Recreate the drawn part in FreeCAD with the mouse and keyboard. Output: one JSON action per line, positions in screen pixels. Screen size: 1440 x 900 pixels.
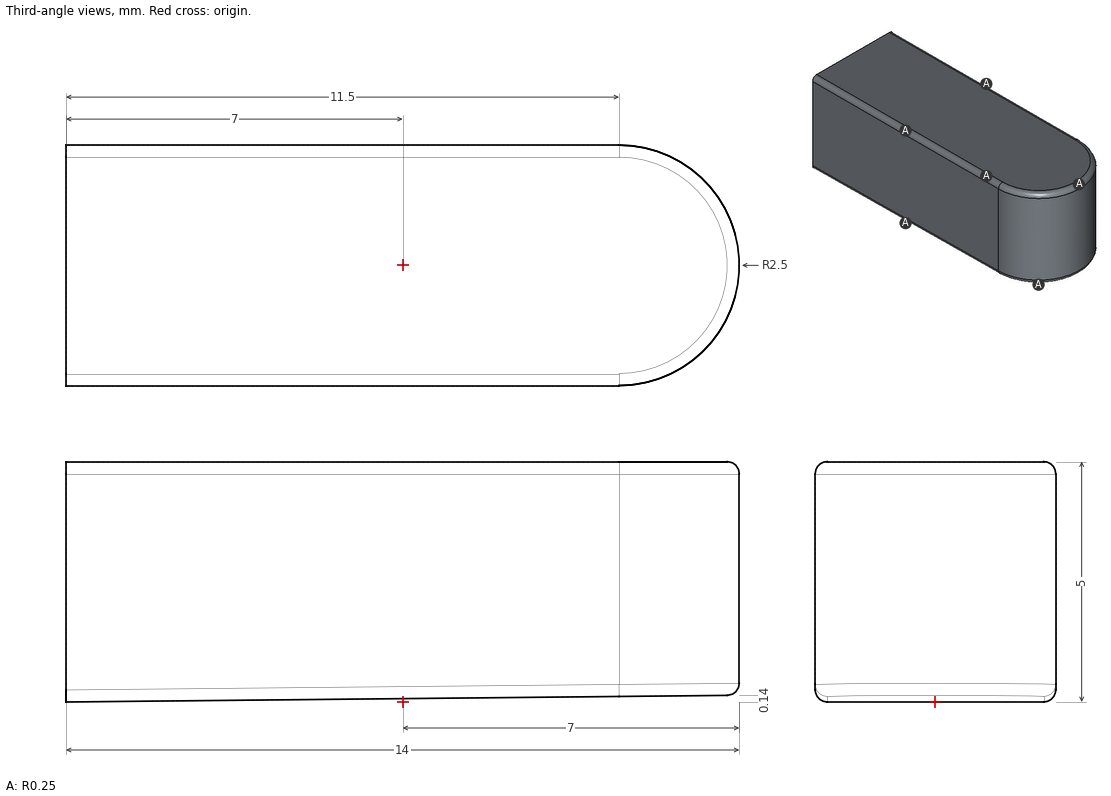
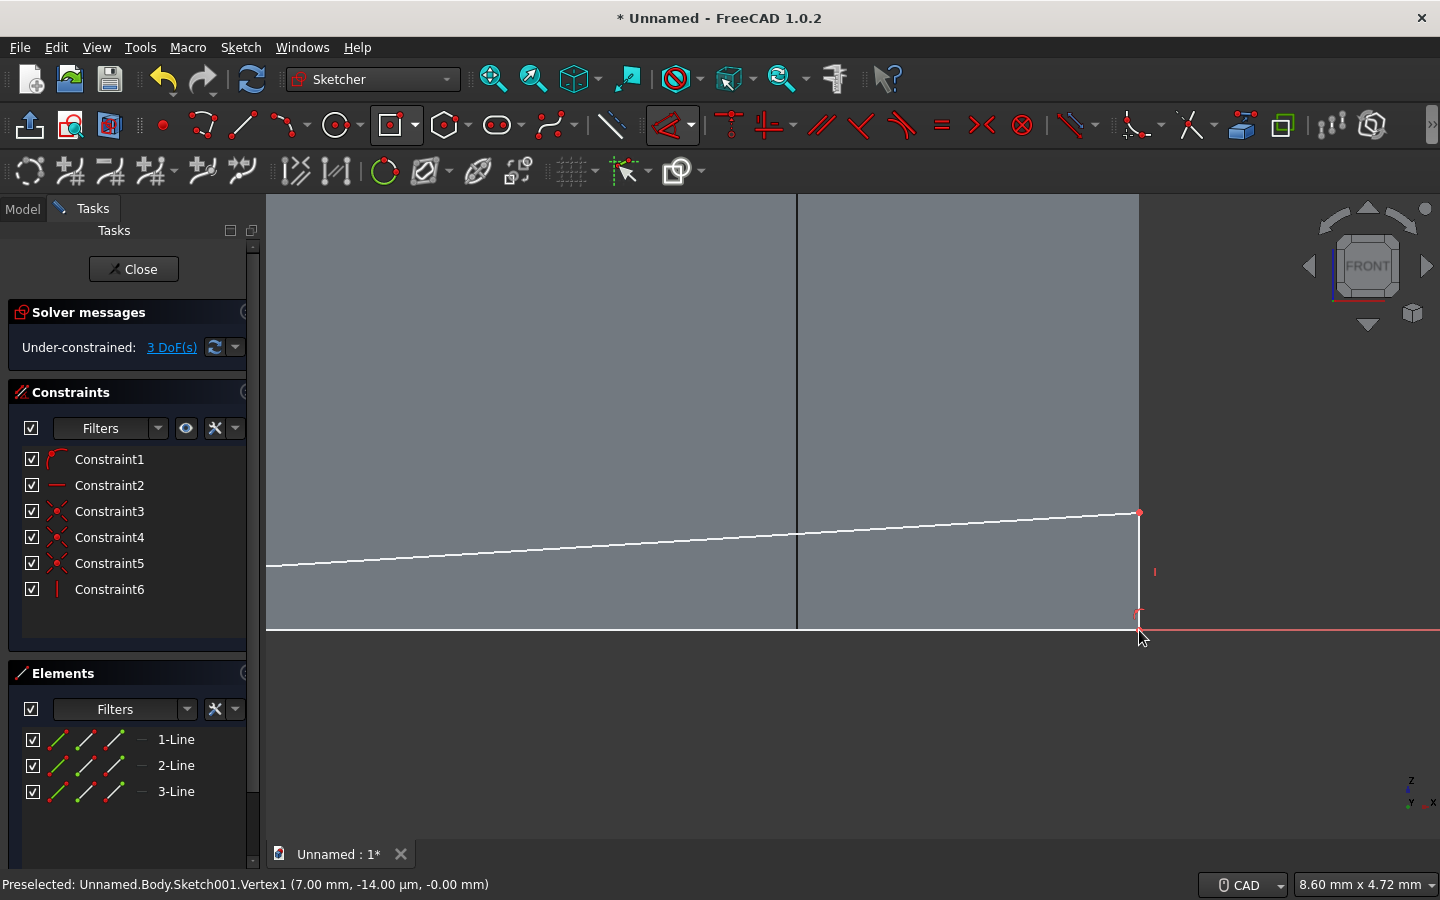
{"action": "left_click", "coordinate": [666, 126]}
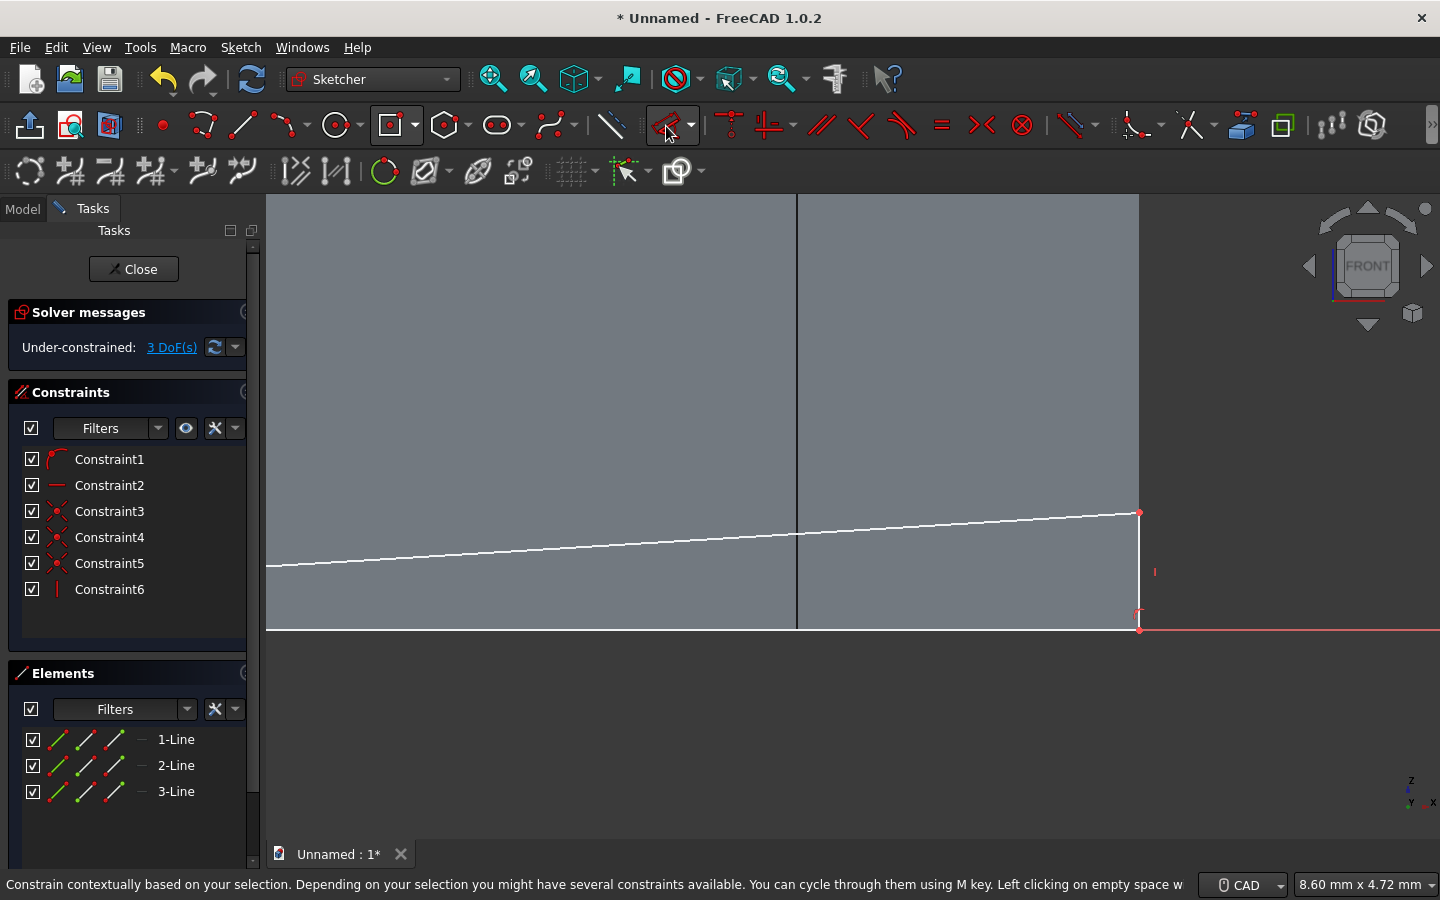
{"action": "left_click", "coordinate": [566, 630]}
{"action": "left_click", "coordinate": [717, 664]}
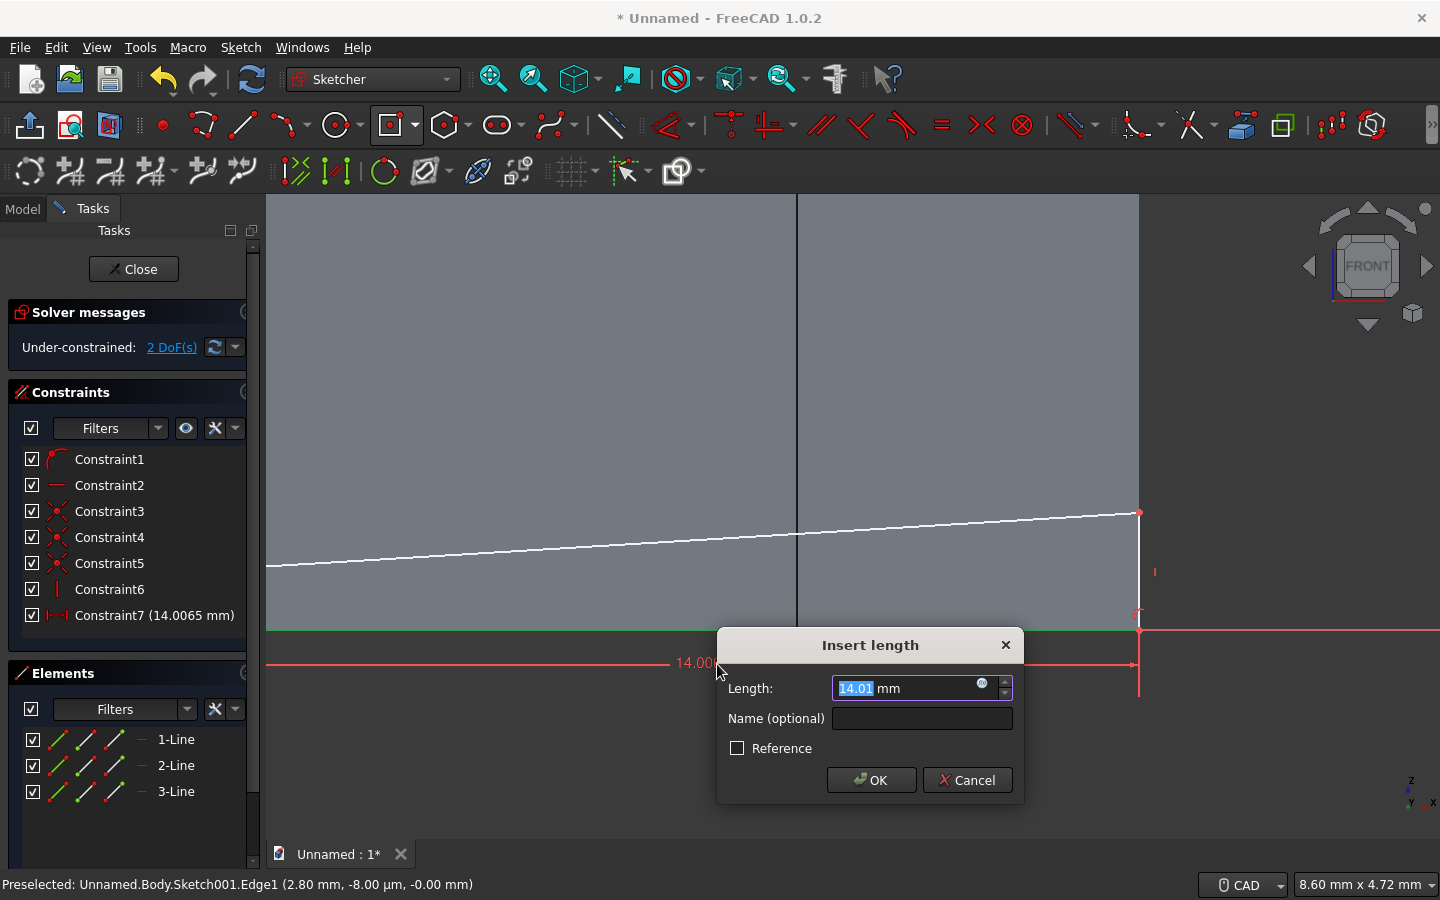
{"action": "type", "text": "14"}
{"action": "key", "text": "Return"}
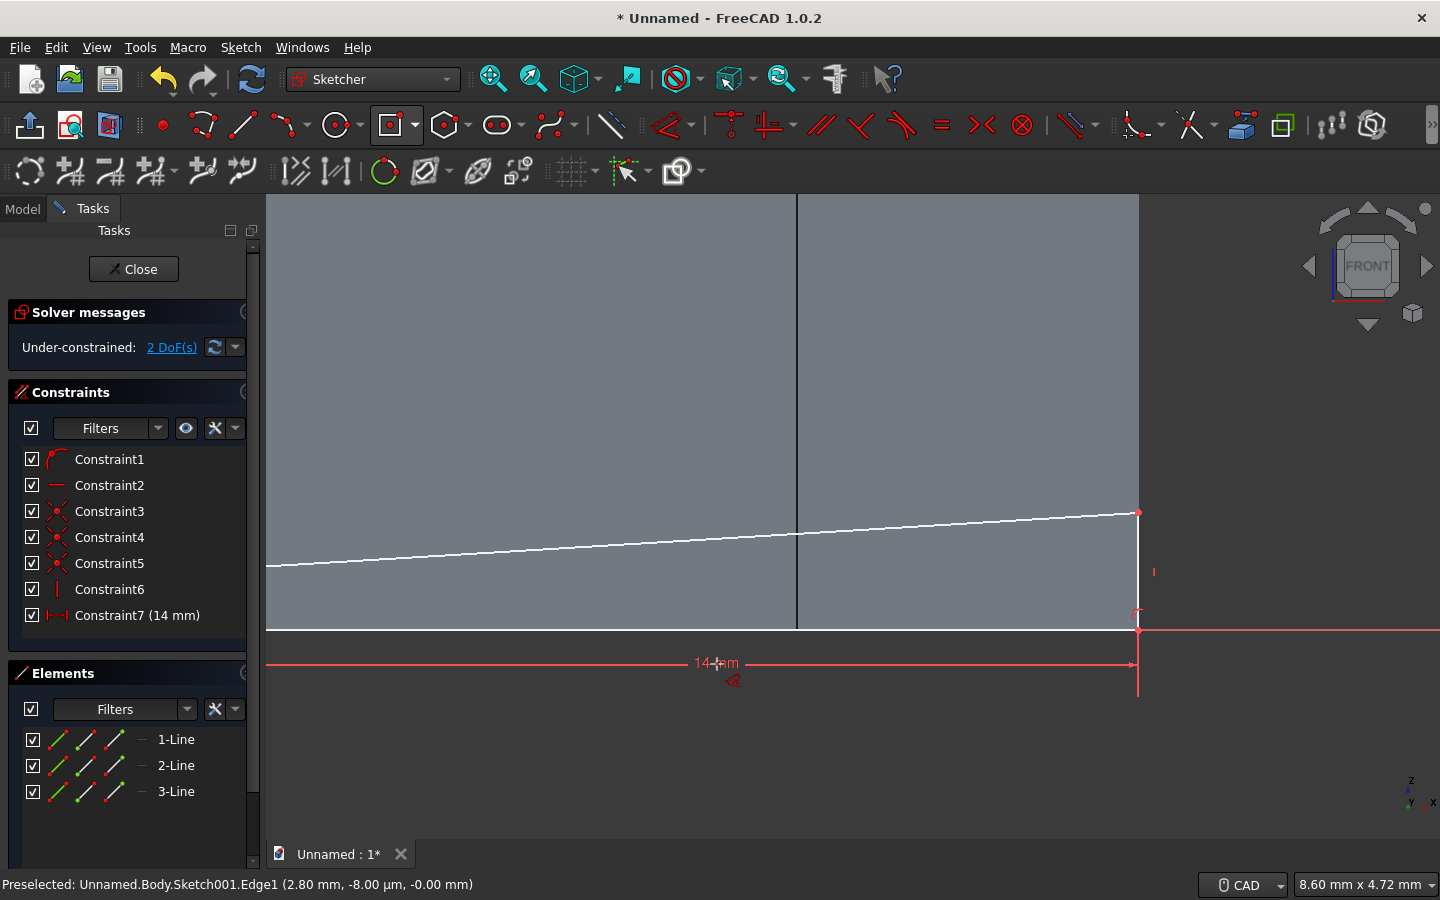
{"action": "left_click", "coordinate": [1138, 630]}
{"action": "left_click", "coordinate": [522, 664]}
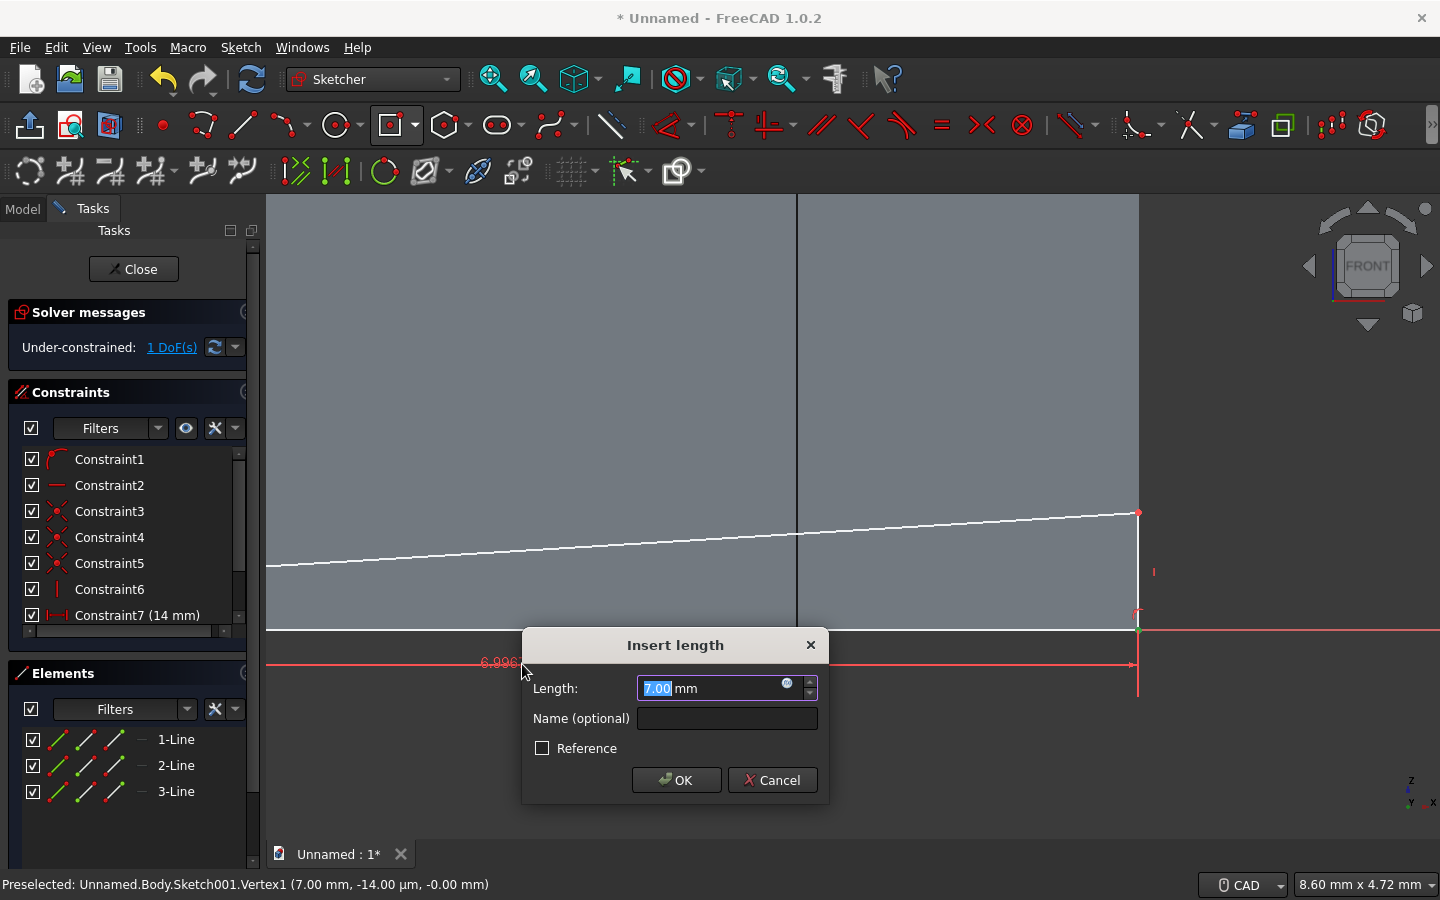
{"action": "type", "text": "7"}
{"action": "key", "text": "Return"}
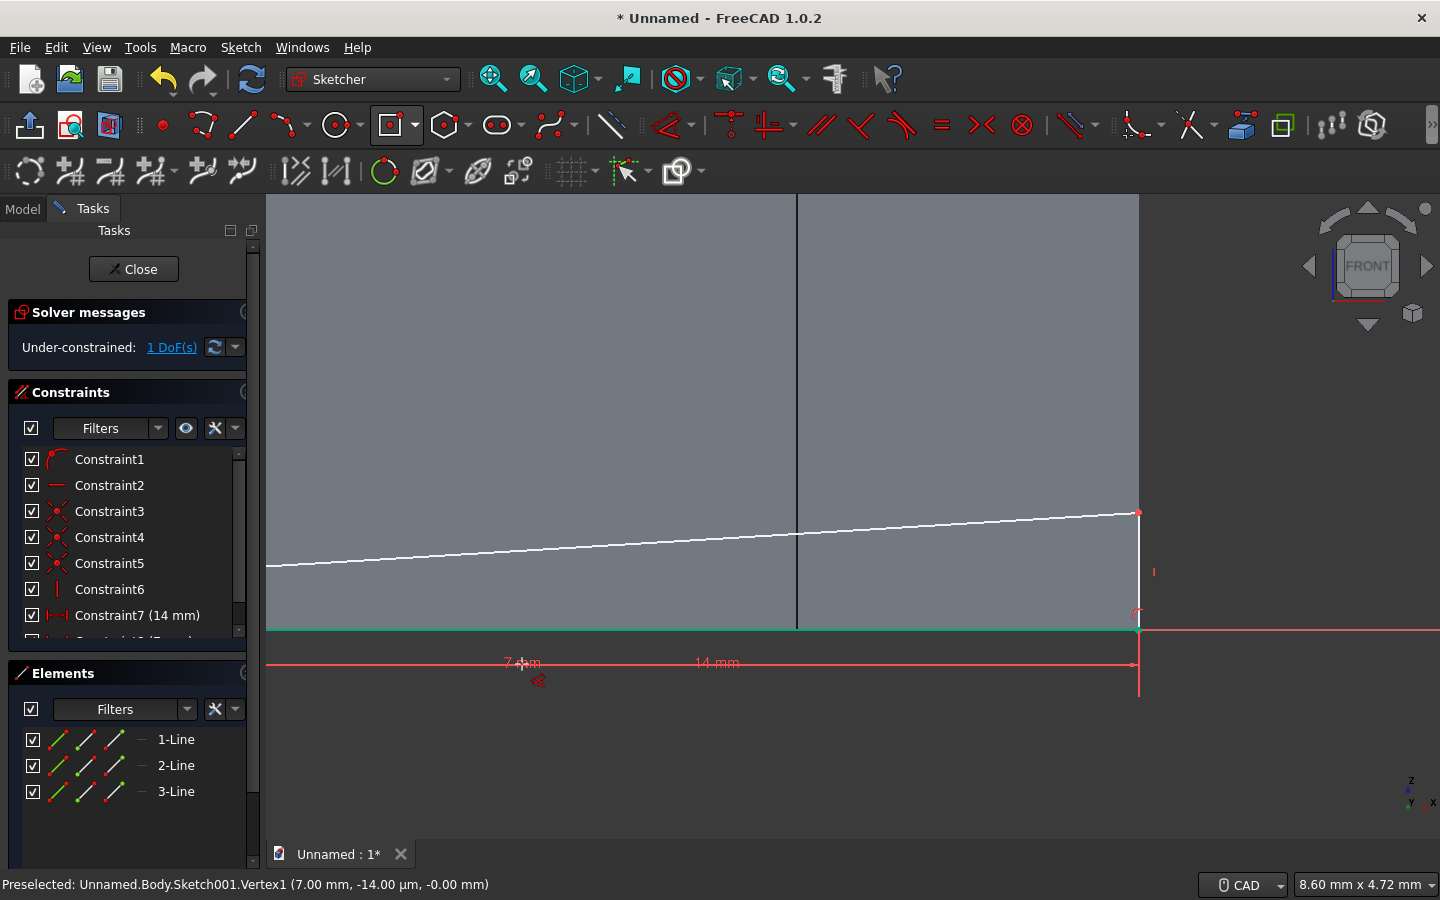
{"action": "scroll", "coordinate": [1139, 548], "scroll_direction": "up", "scroll_amount": 4}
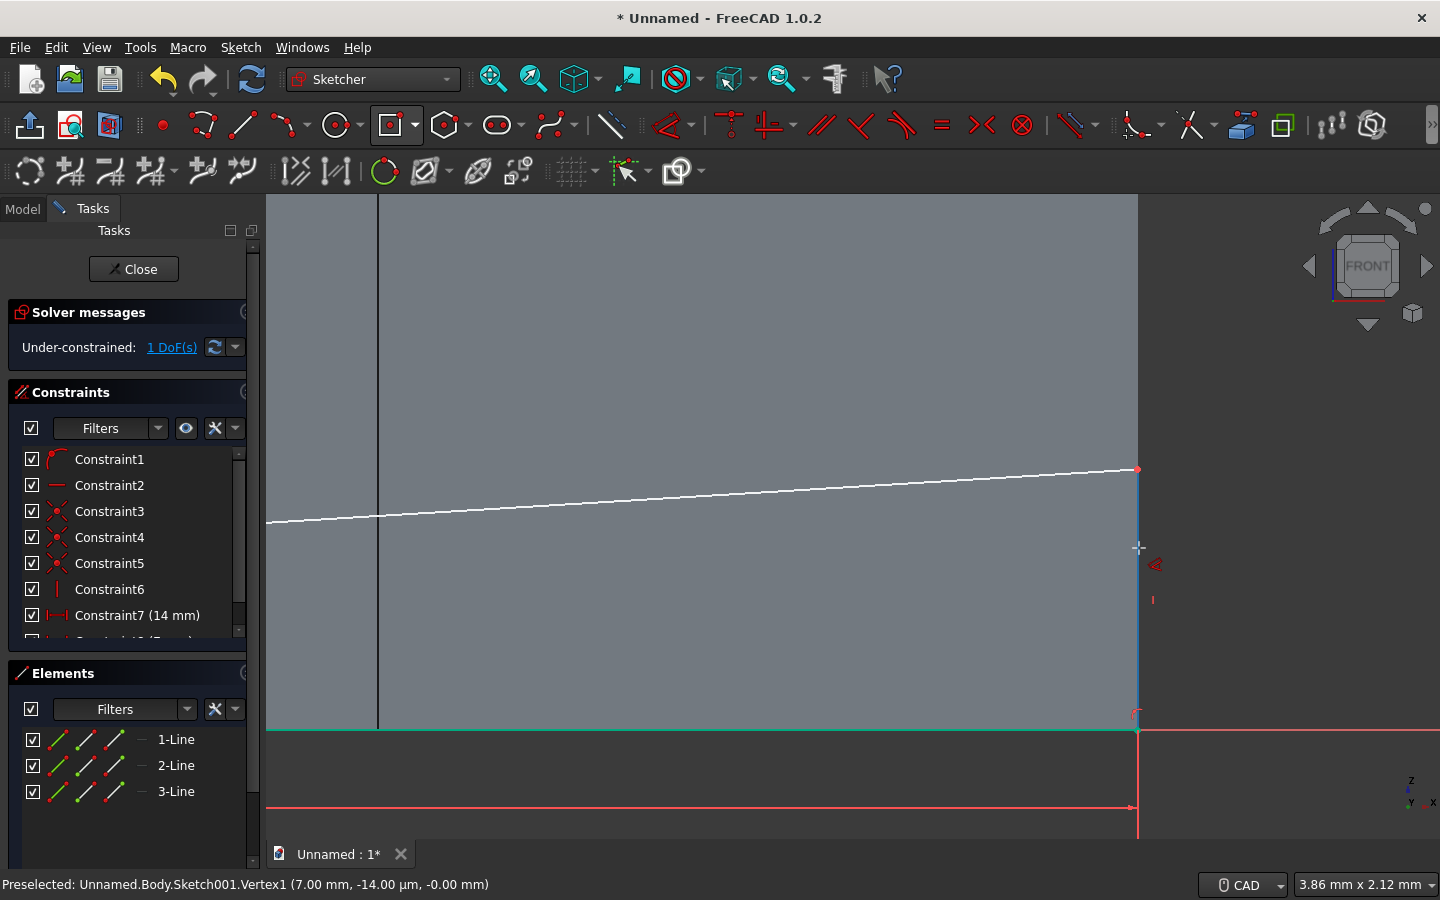
{"action": "left_click", "coordinate": [1138, 548]}
{"action": "left_click", "coordinate": [1172, 600]}